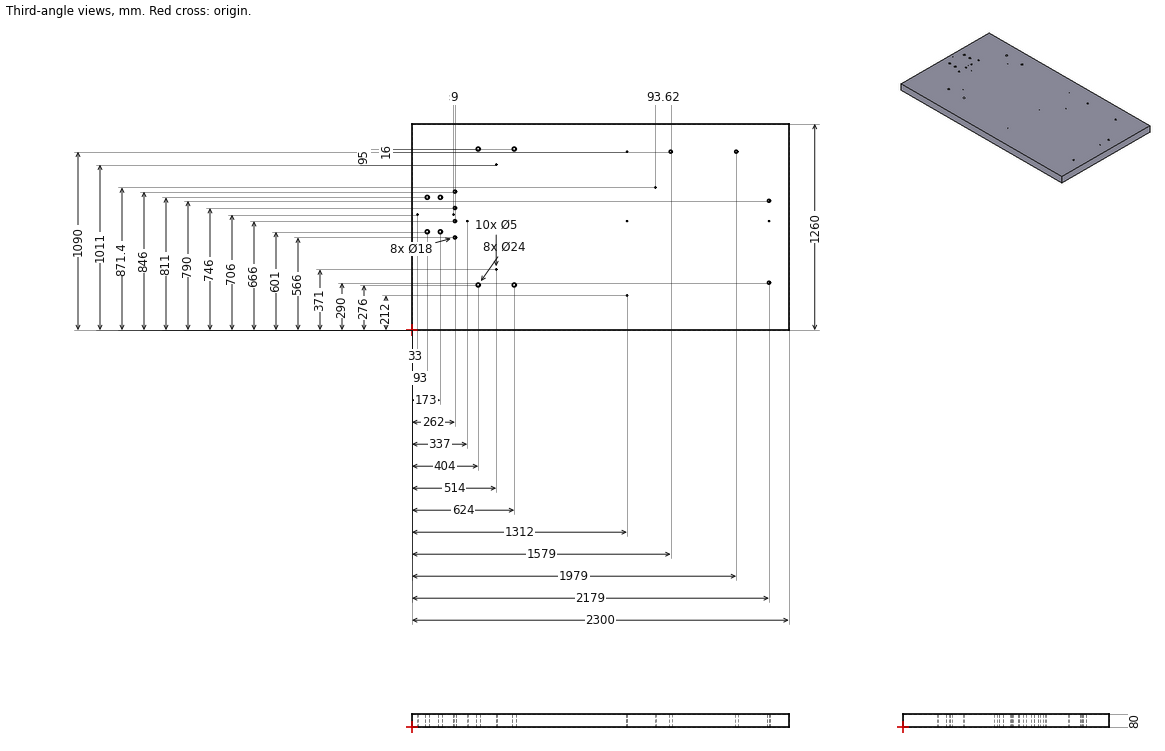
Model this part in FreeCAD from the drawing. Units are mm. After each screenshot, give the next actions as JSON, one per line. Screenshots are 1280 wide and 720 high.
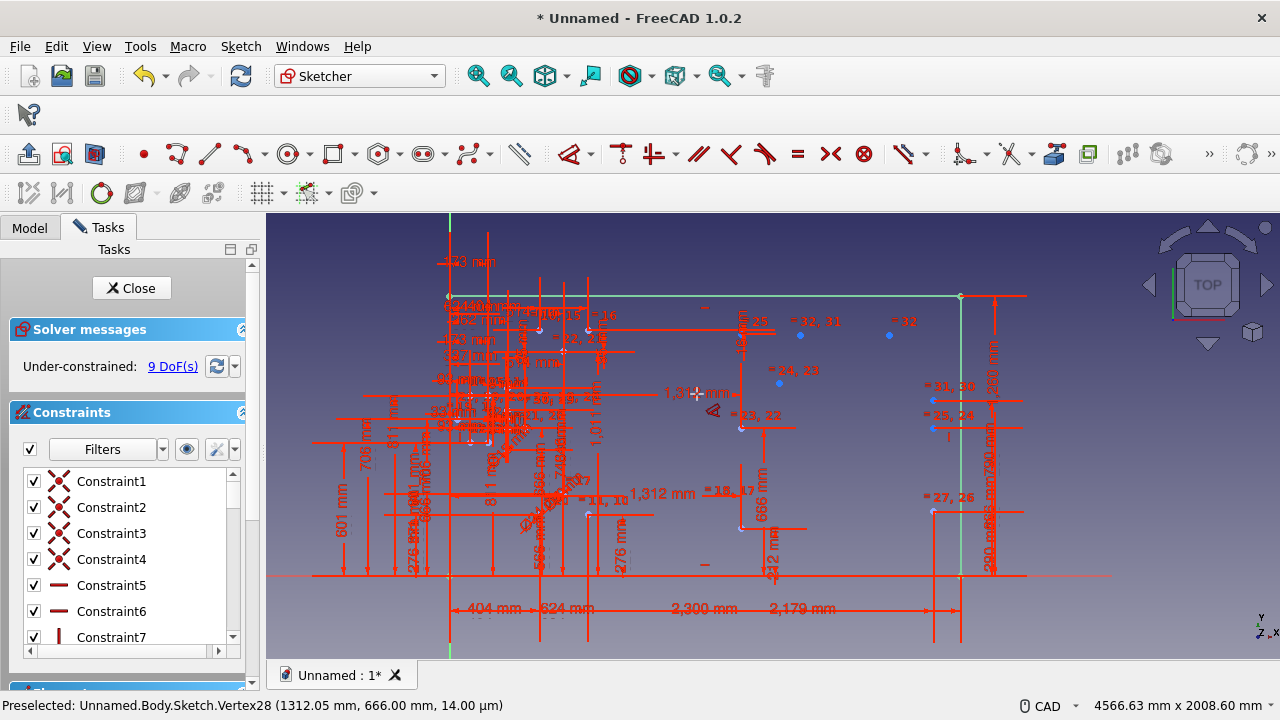
{"action": "left_click", "coordinate": [934, 428]}
{"action": "left_click", "coordinate": [803, 394]}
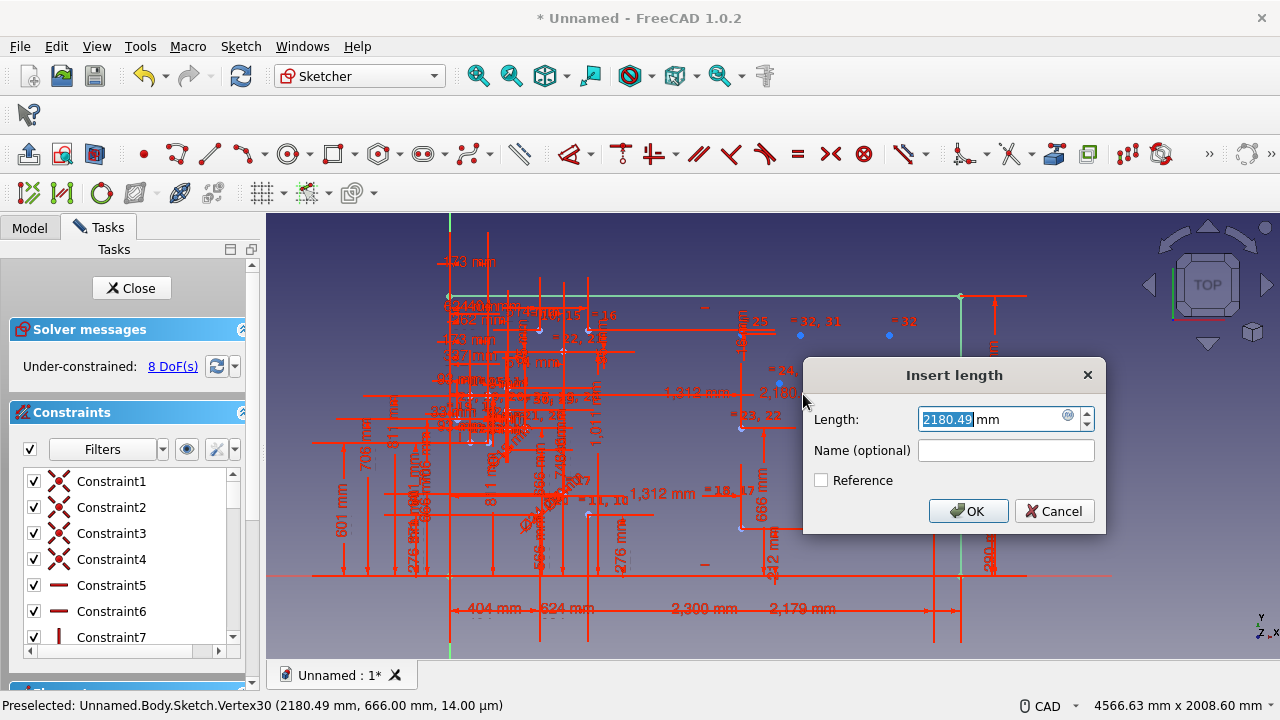
{"action": "type", "text": "2179"}
{"action": "key", "text": "Return"}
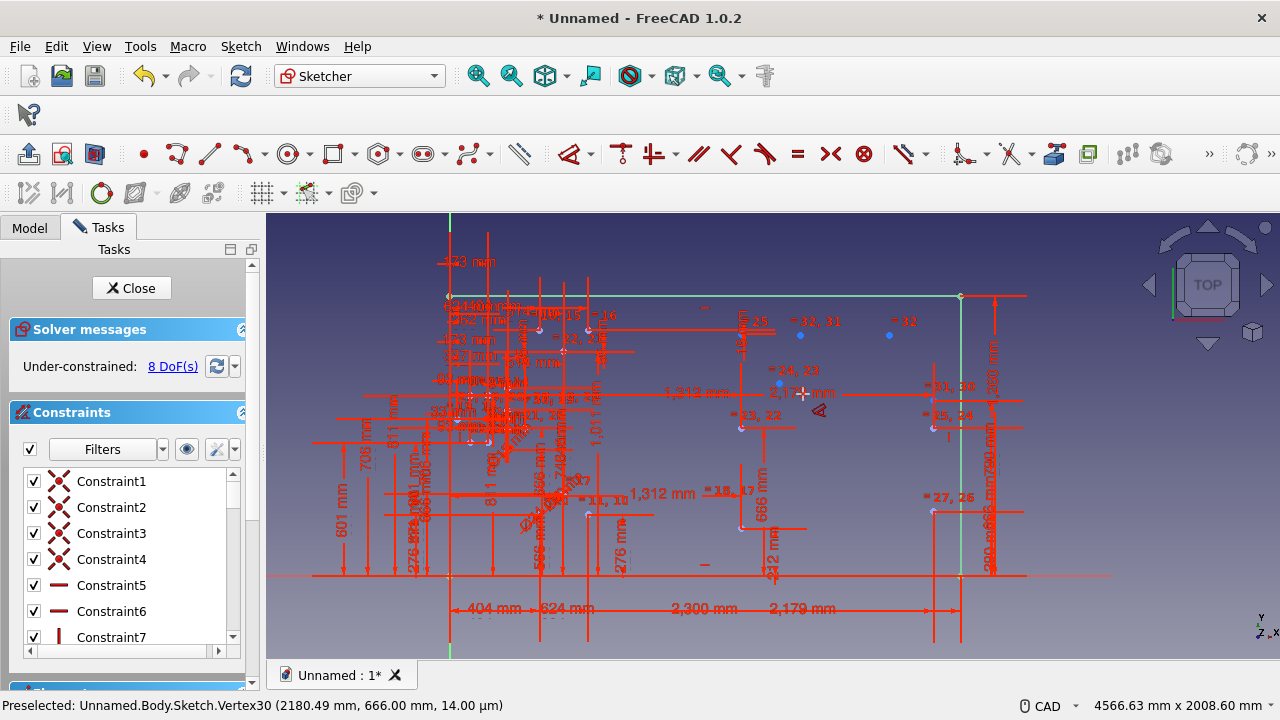
{"action": "left_click", "coordinate": [934, 401]}
{"action": "left_click", "coordinate": [692, 367]}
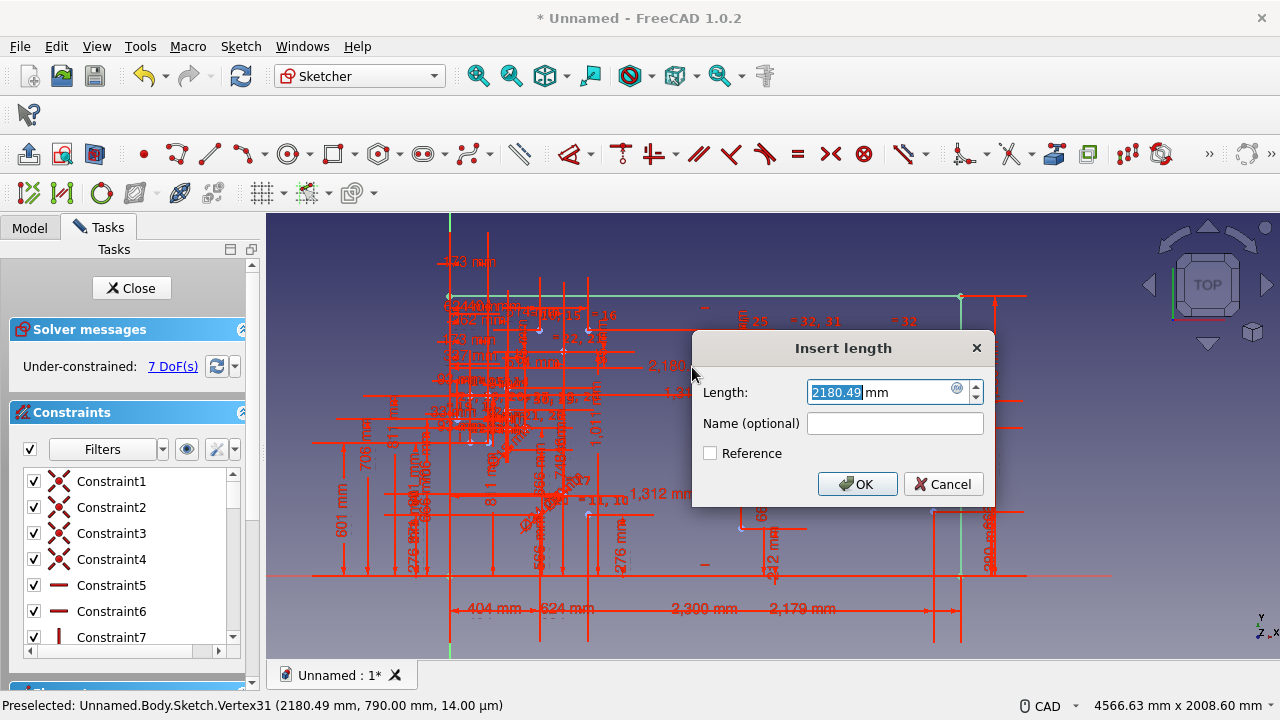
{"action": "type", "text": "2179"}
{"action": "key", "text": "Return"}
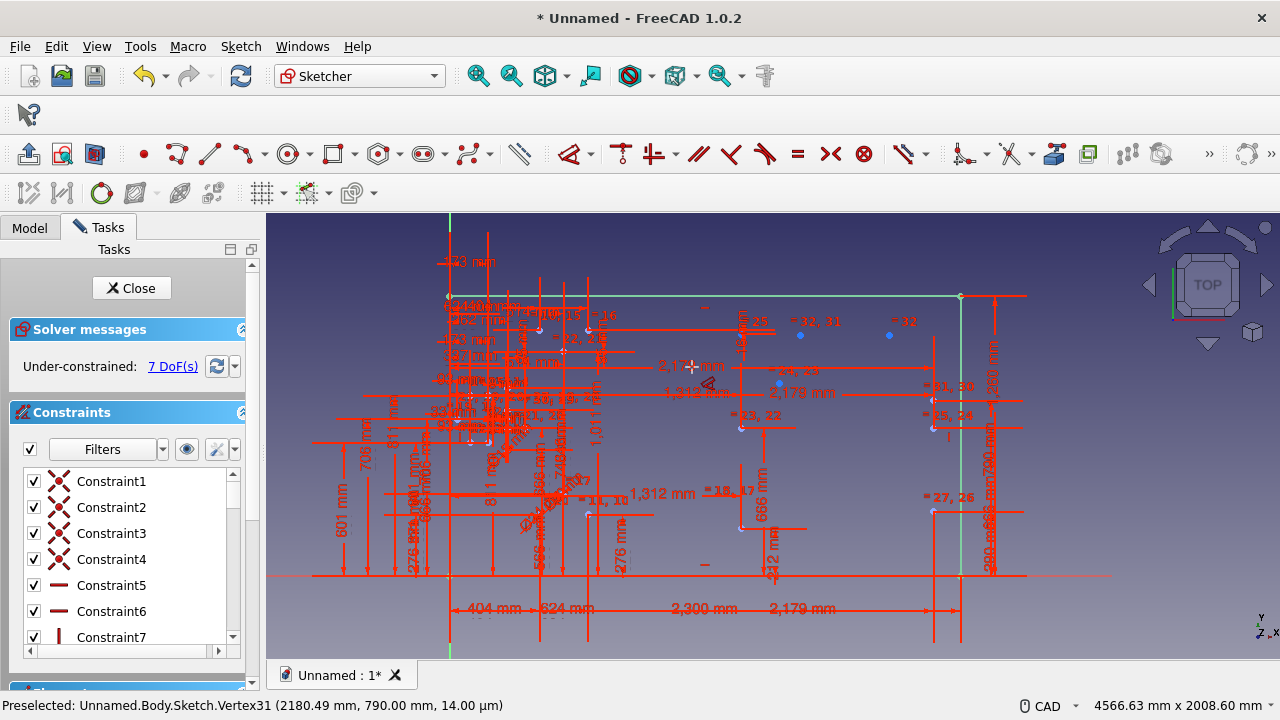
{"action": "left_click", "coordinate": [741, 334]}
{"action": "left_click", "coordinate": [596, 276]}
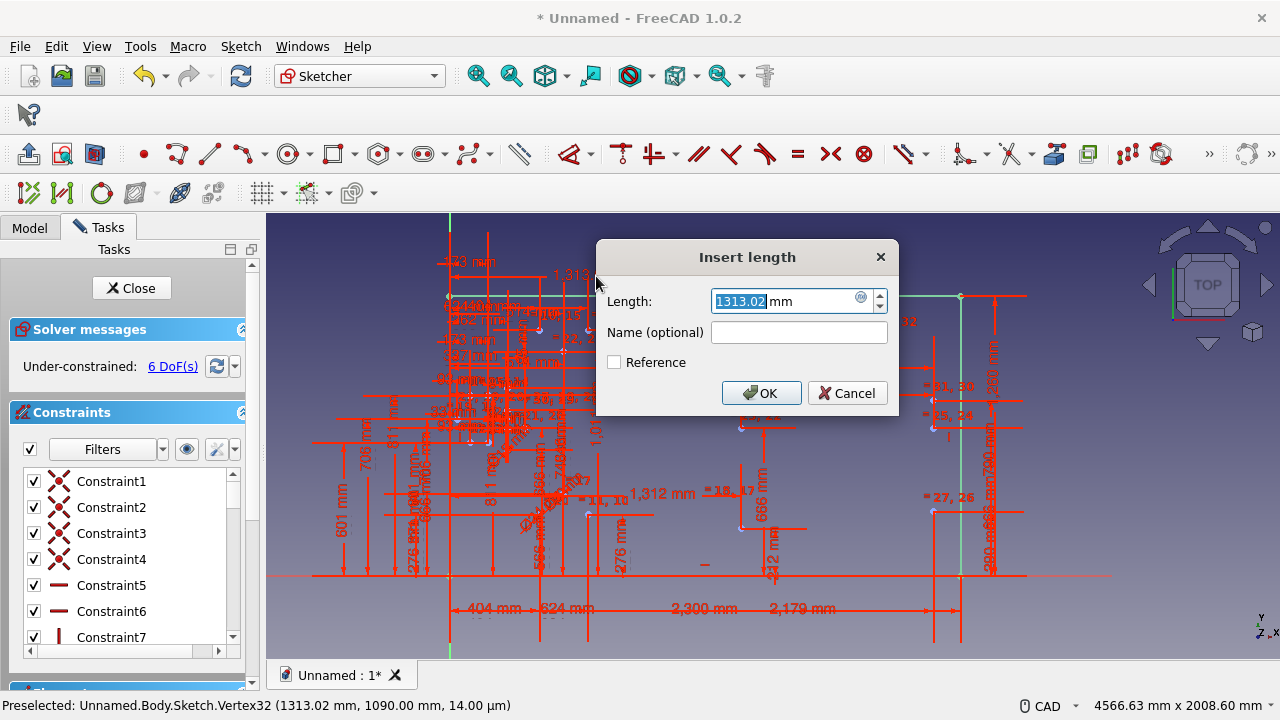
{"action": "type", "text": "1312"}
{"action": "key", "text": "Return"}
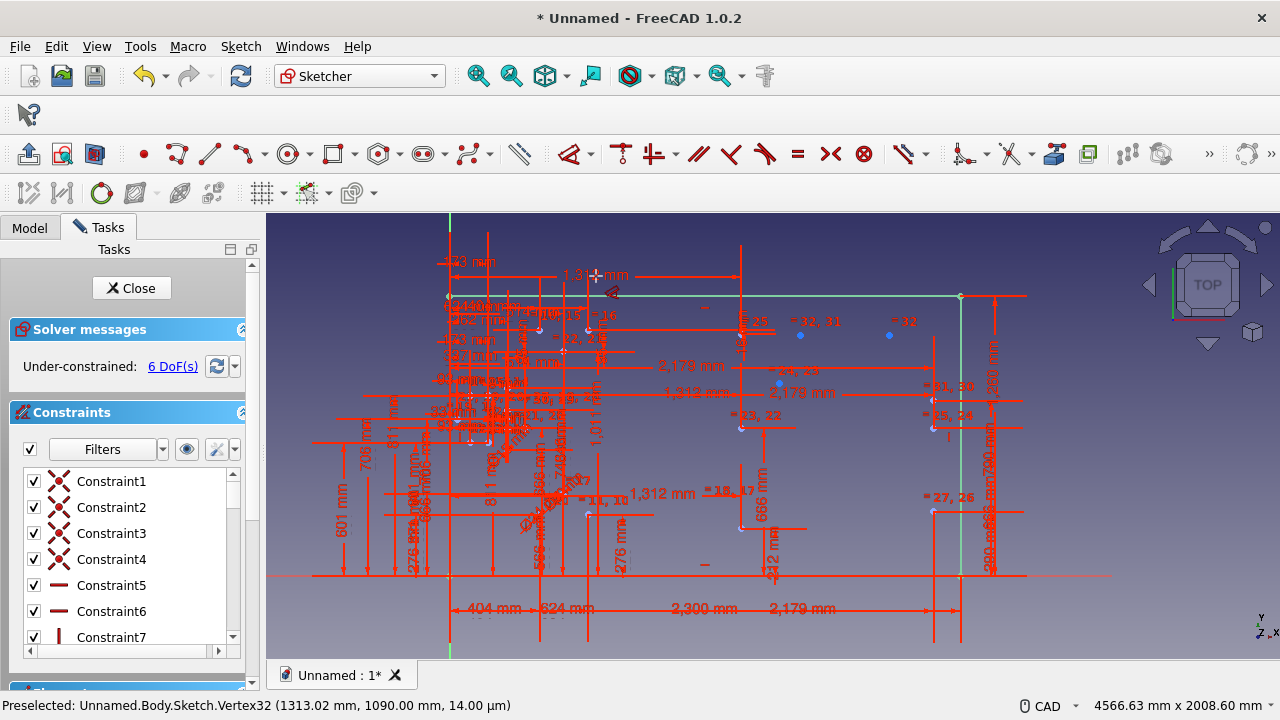
{"action": "left_click", "coordinate": [800, 335]}
{"action": "left_click", "coordinate": [706, 277]}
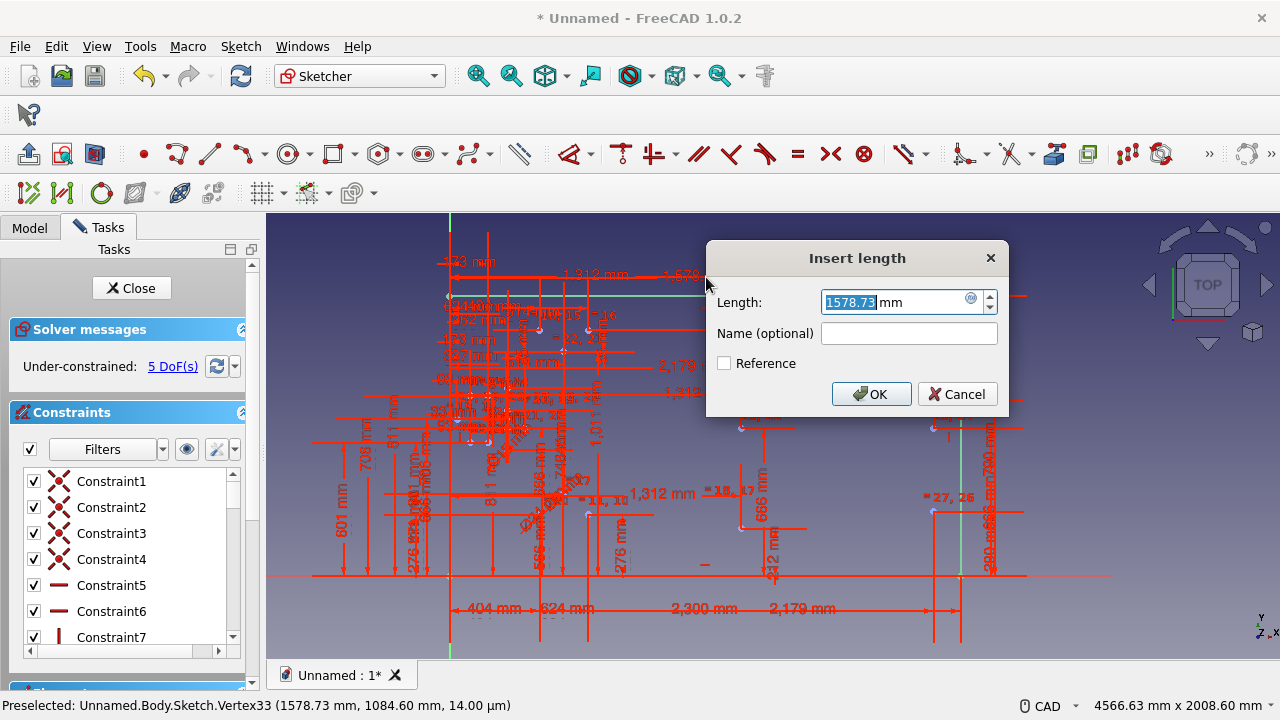
{"action": "type", "text": "1579"}
{"action": "key", "text": "Return"}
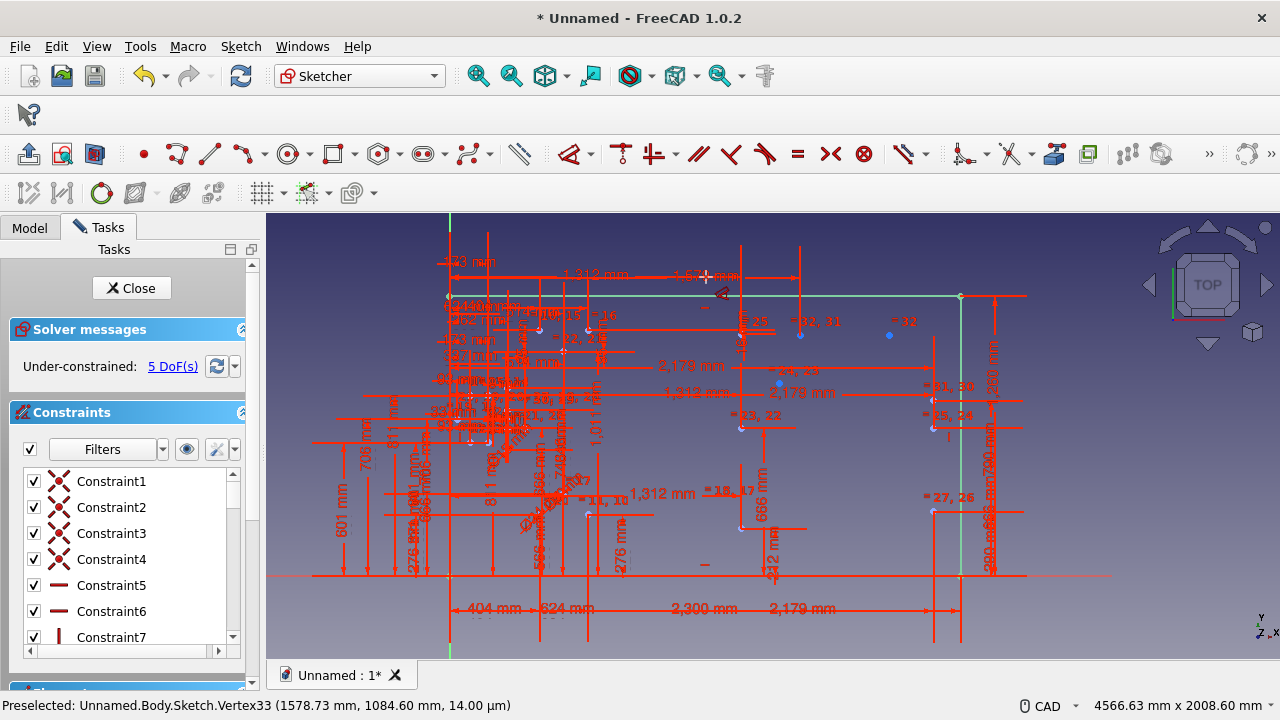
{"action": "left_click", "coordinate": [800, 335]}
{"action": "left_click", "coordinate": [834, 456]}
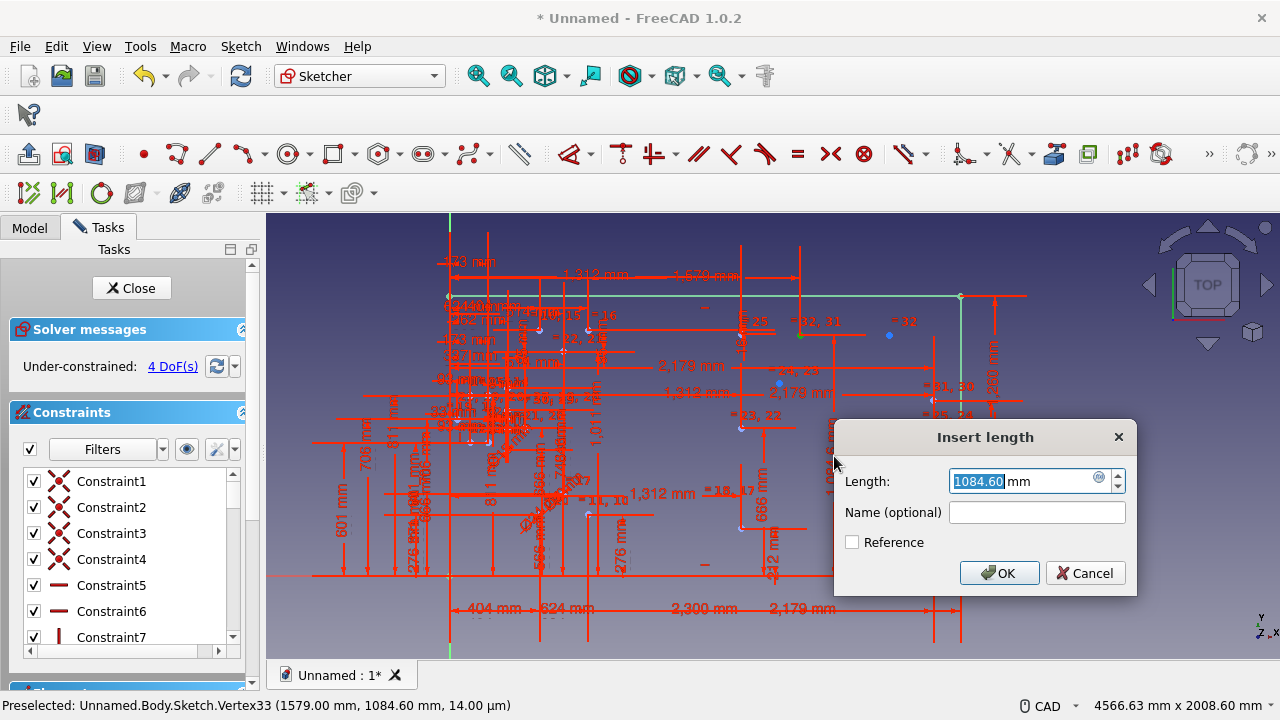
{"action": "type", "text": "1090"}
{"action": "key", "text": "Return"}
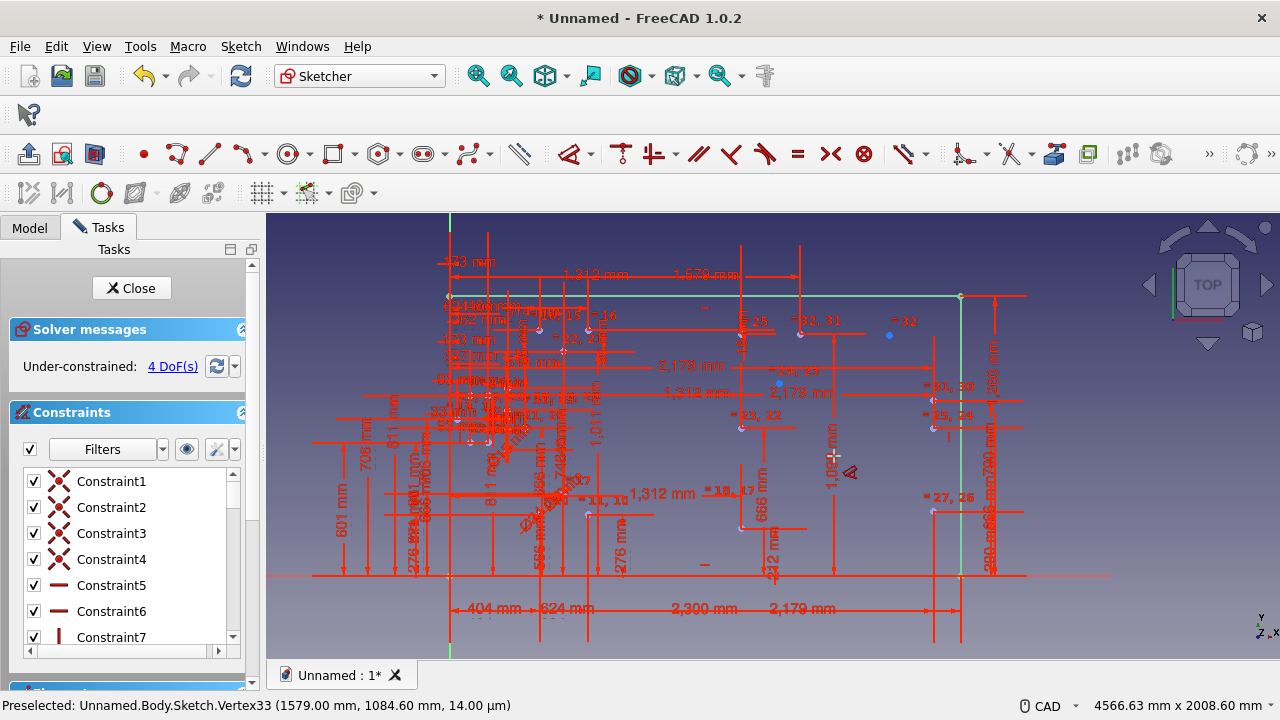
{"action": "left_click", "coordinate": [889, 335]}
{"action": "left_click", "coordinate": [823, 277]}